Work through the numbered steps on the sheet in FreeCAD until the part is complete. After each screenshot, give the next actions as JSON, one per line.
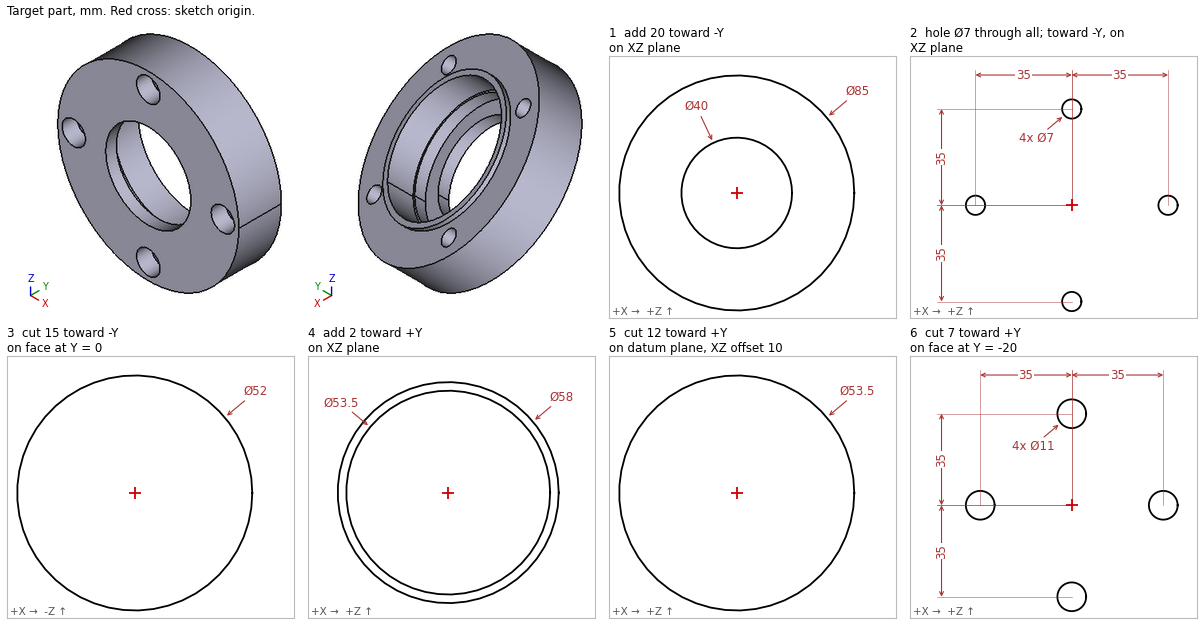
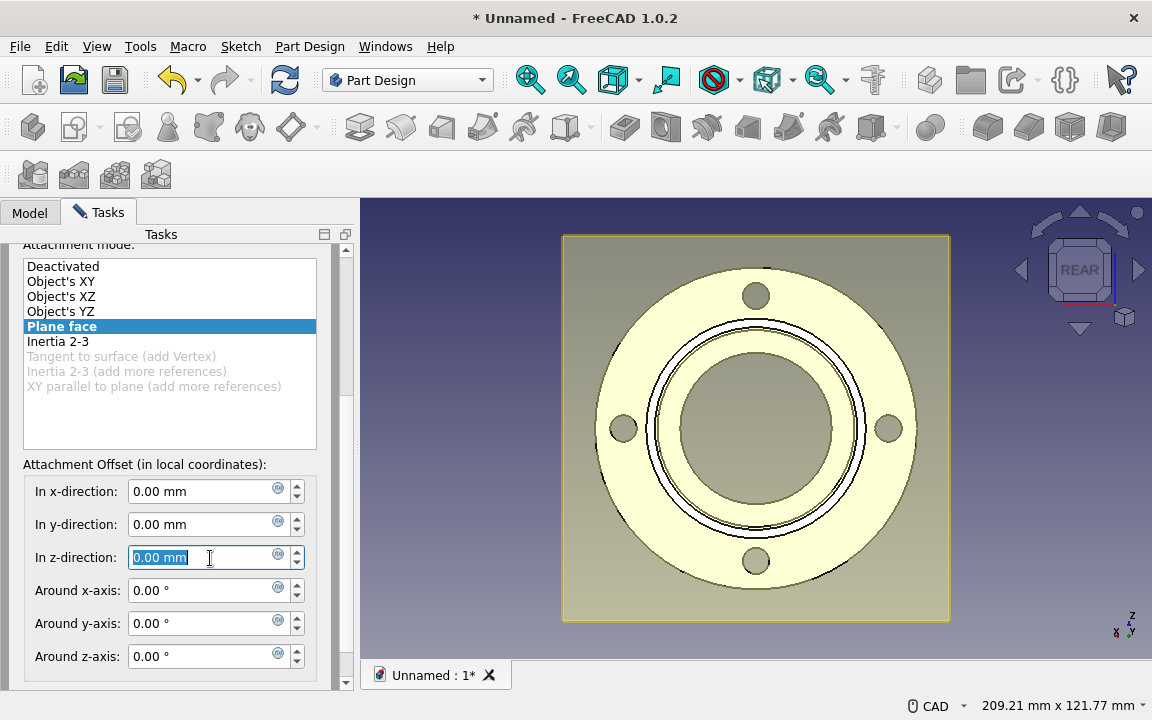
{"action": "type", "text": "10"}
{"action": "key", "text": "Tab"}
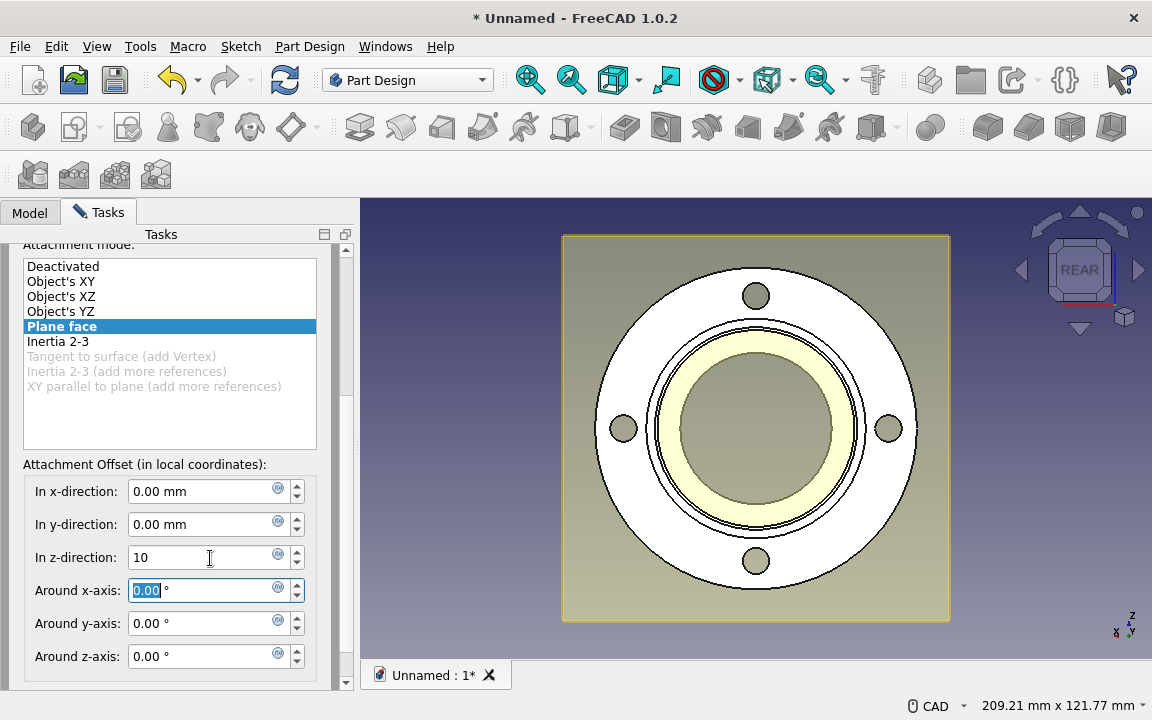
{"action": "scroll", "coordinate": [346, 467], "scroll_direction": "up", "scroll_amount": 5}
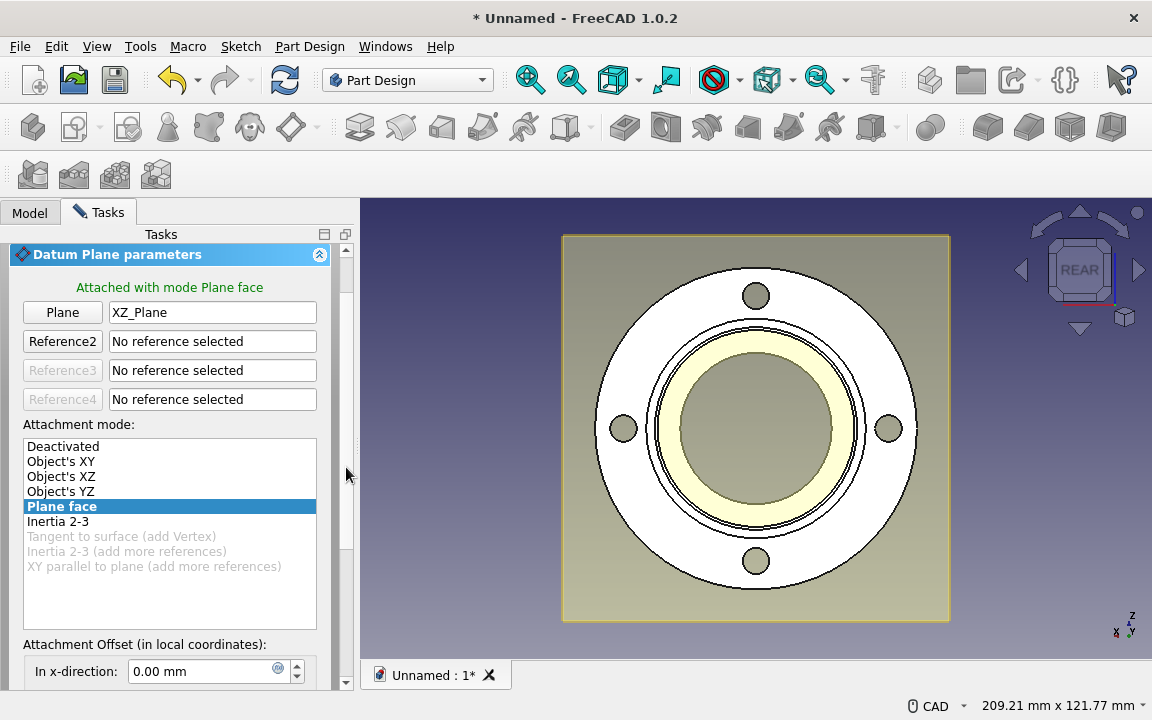
{"action": "left_click", "coordinate": [127, 273]}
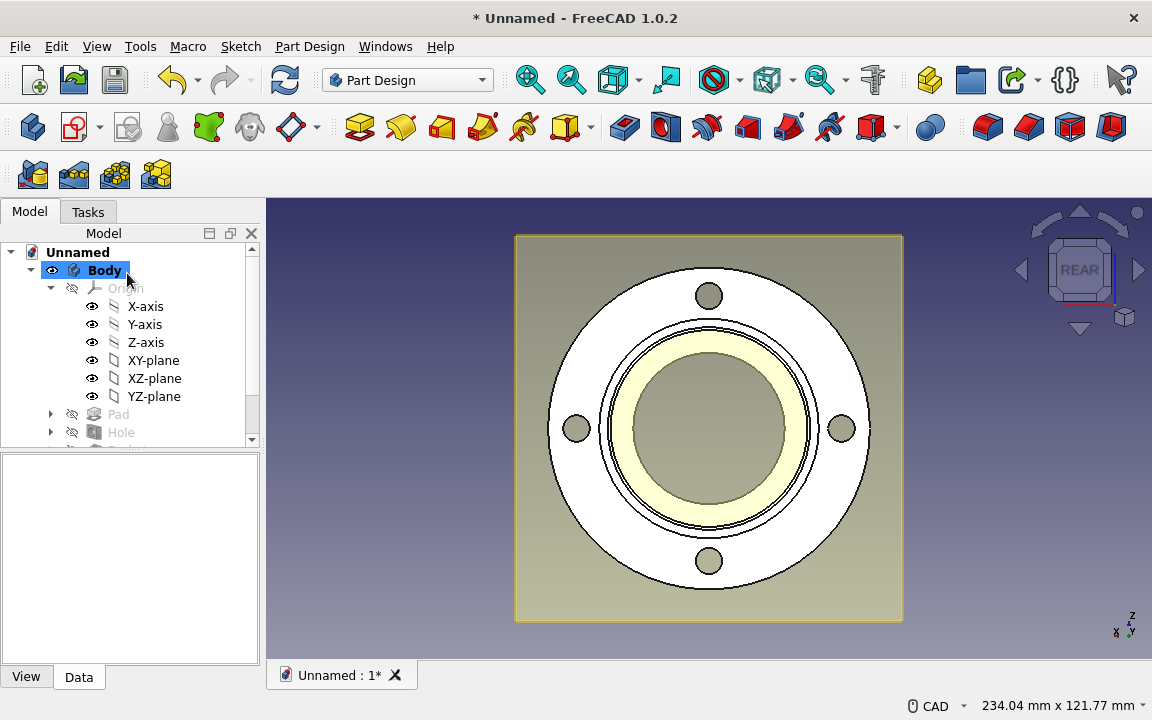
{"action": "scroll", "coordinate": [101, 338], "scroll_direction": "down", "scroll_amount": 3}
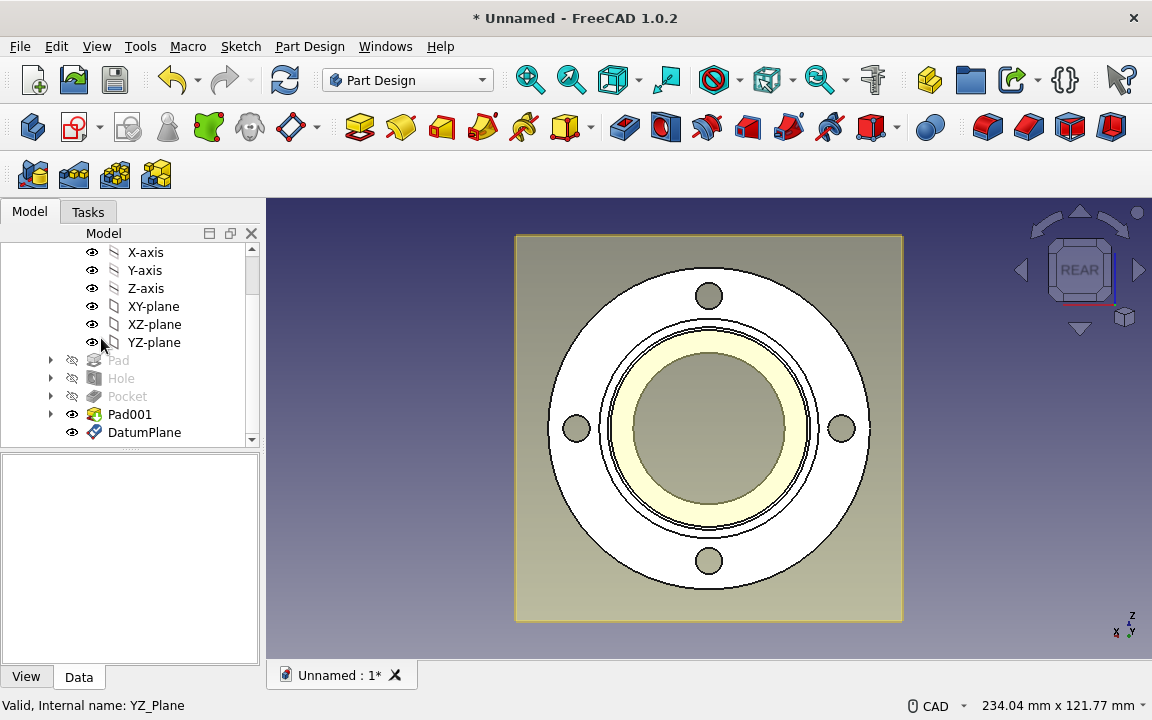
{"action": "left_click", "coordinate": [117, 432]}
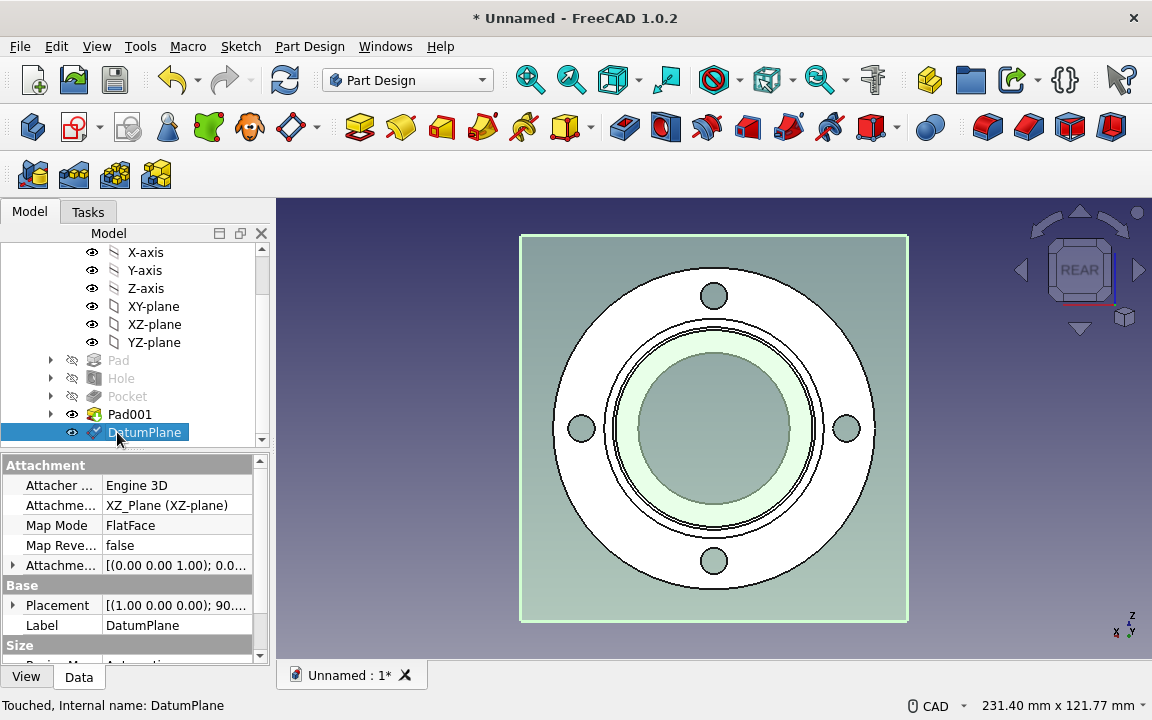
{"action": "left_click", "coordinate": [74, 128]}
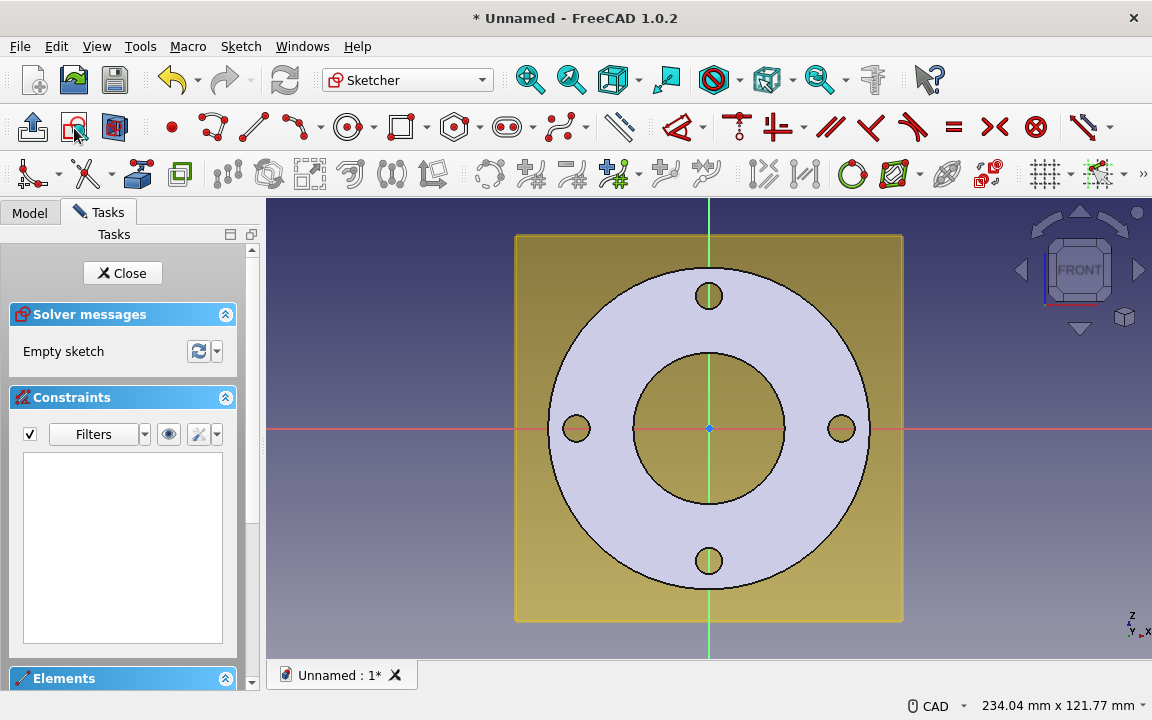
{"action": "key", "text": "q s"}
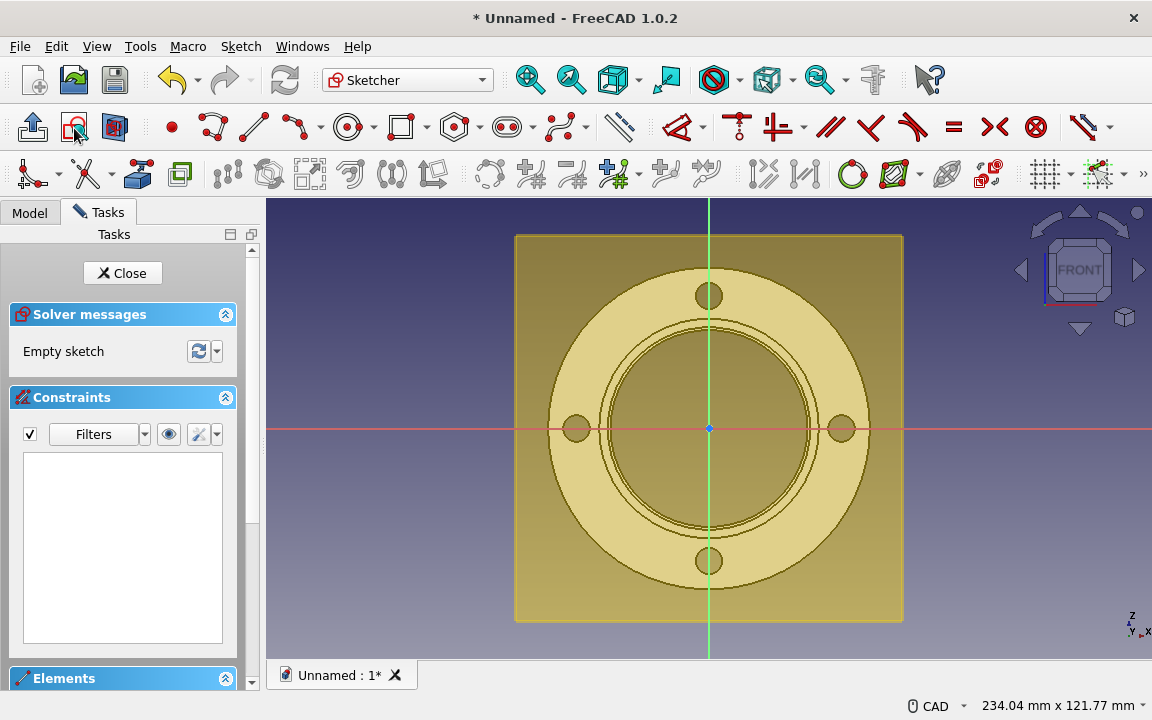
{"action": "scroll", "coordinate": [848, 429], "scroll_direction": "up", "scroll_amount": 2}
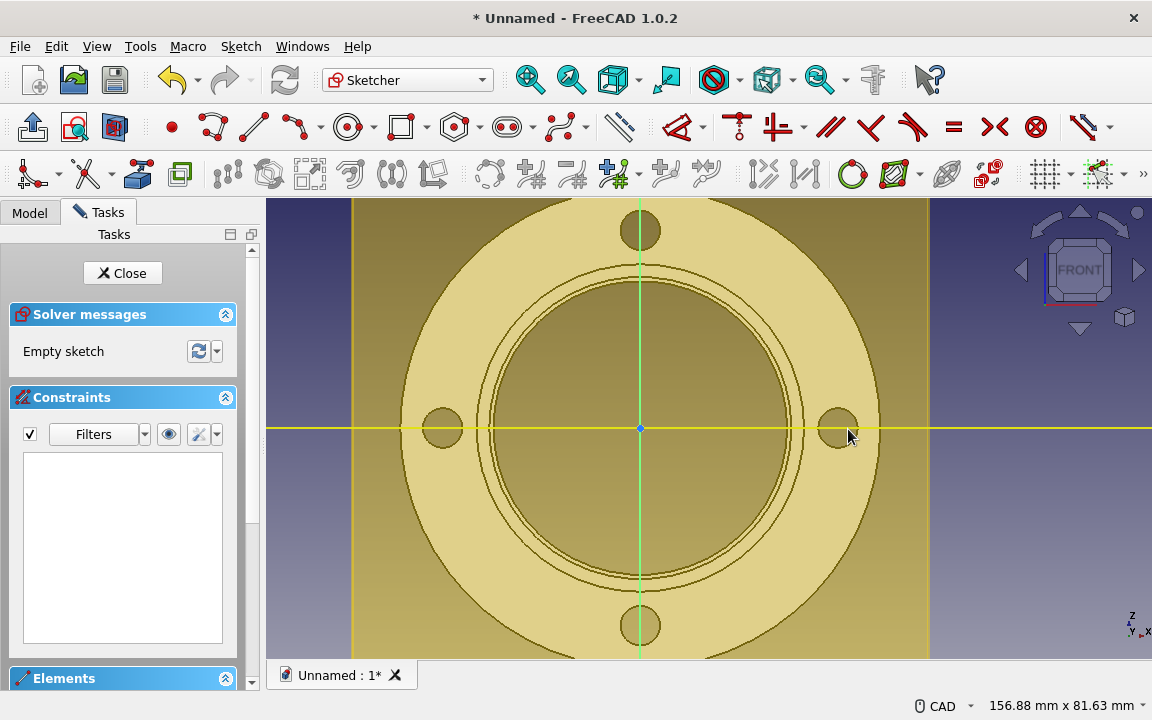
{"action": "left_click", "coordinate": [348, 128]}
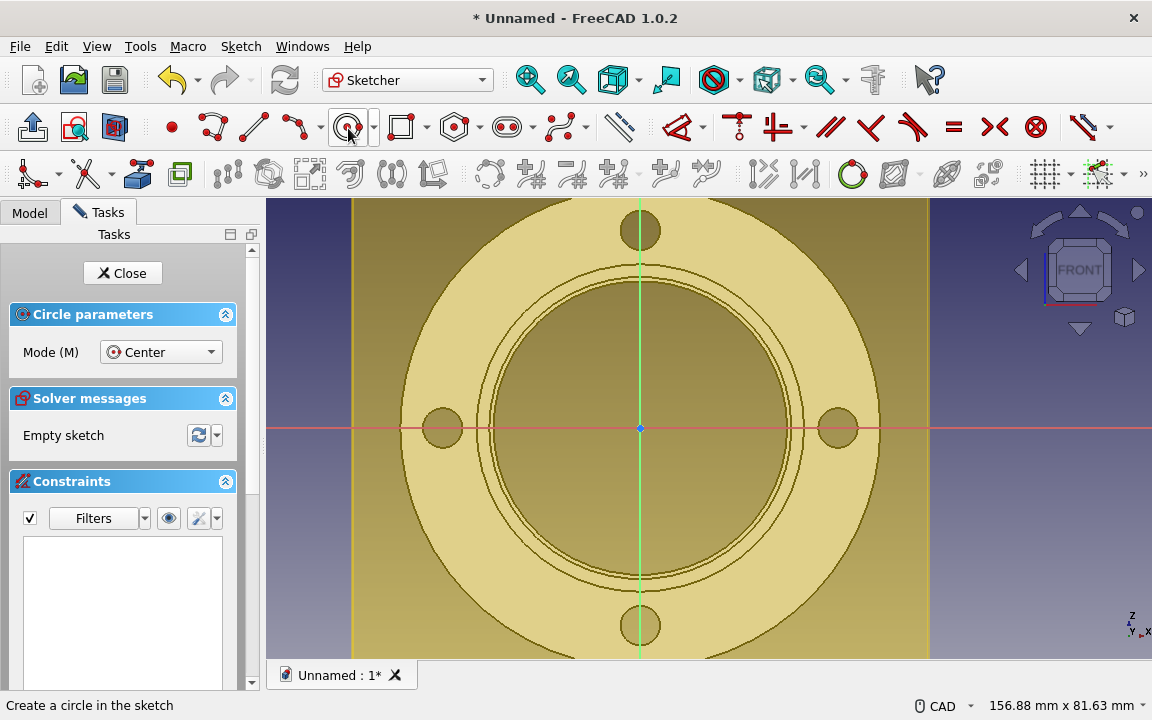
{"action": "left_click", "coordinate": [640, 428]}
{"action": "mouse_move", "coordinate": [747, 321]}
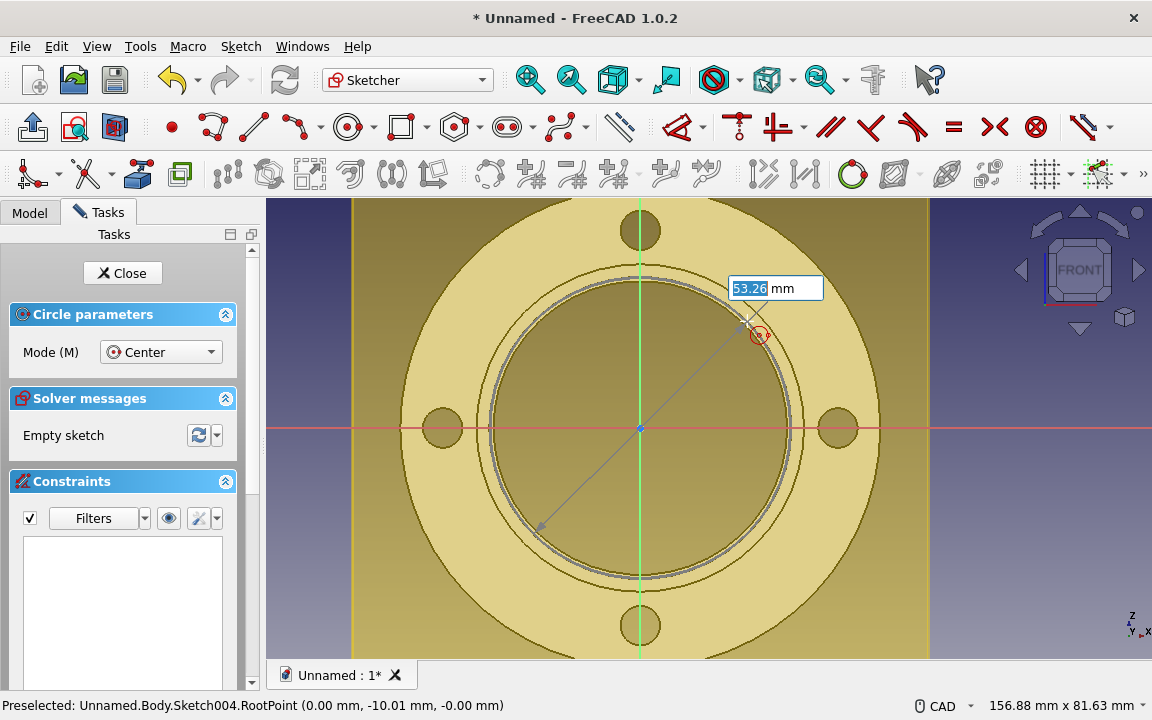
{"action": "type", "text": "53.5"}
{"action": "key", "text": "Return"}
{"action": "key", "text": "Escape"}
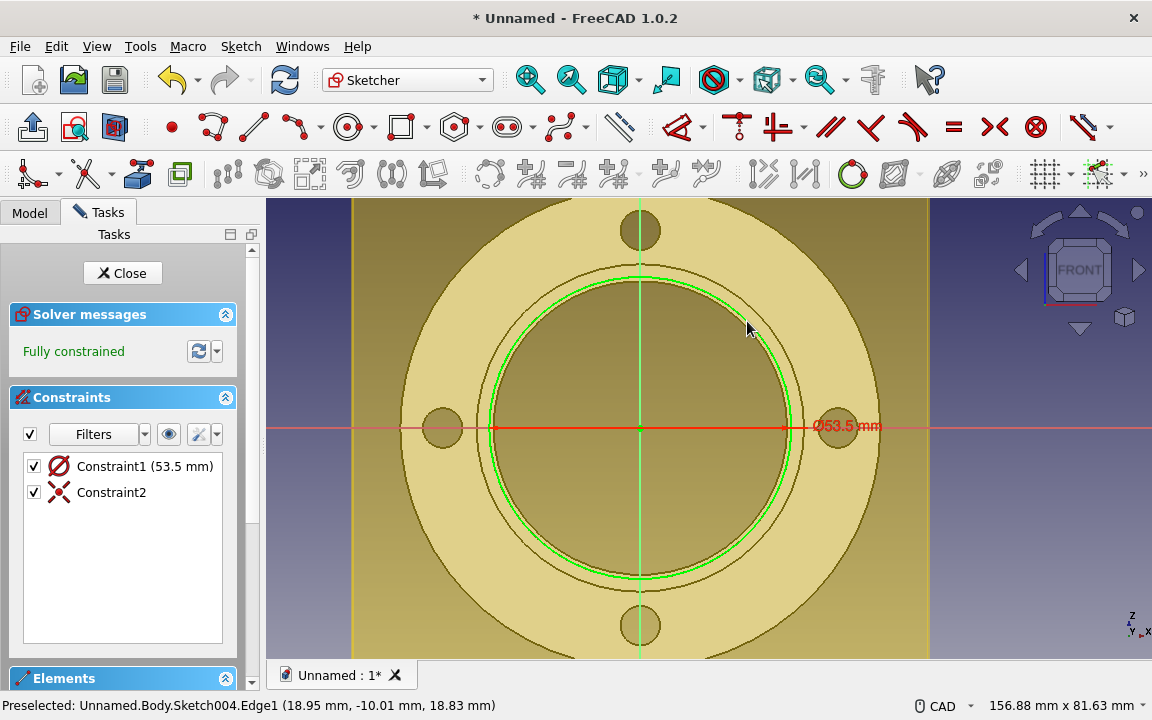
{"action": "left_click", "coordinate": [123, 273]}